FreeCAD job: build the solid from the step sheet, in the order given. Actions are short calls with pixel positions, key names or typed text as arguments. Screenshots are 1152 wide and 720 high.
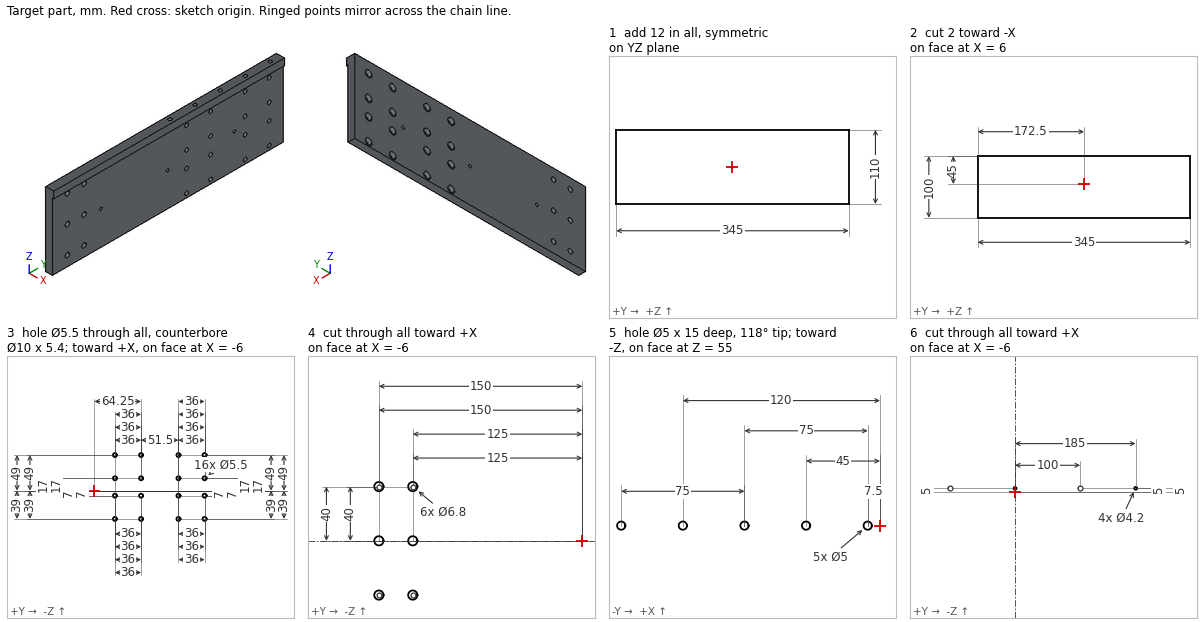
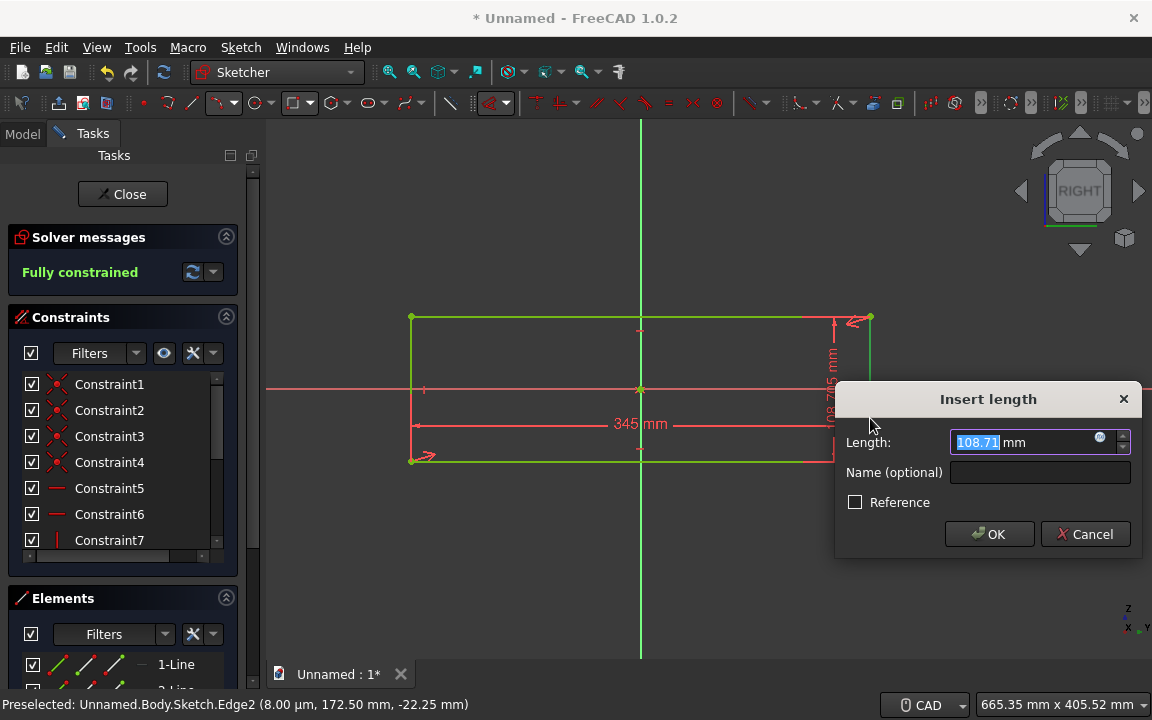
text(110)
key(Return)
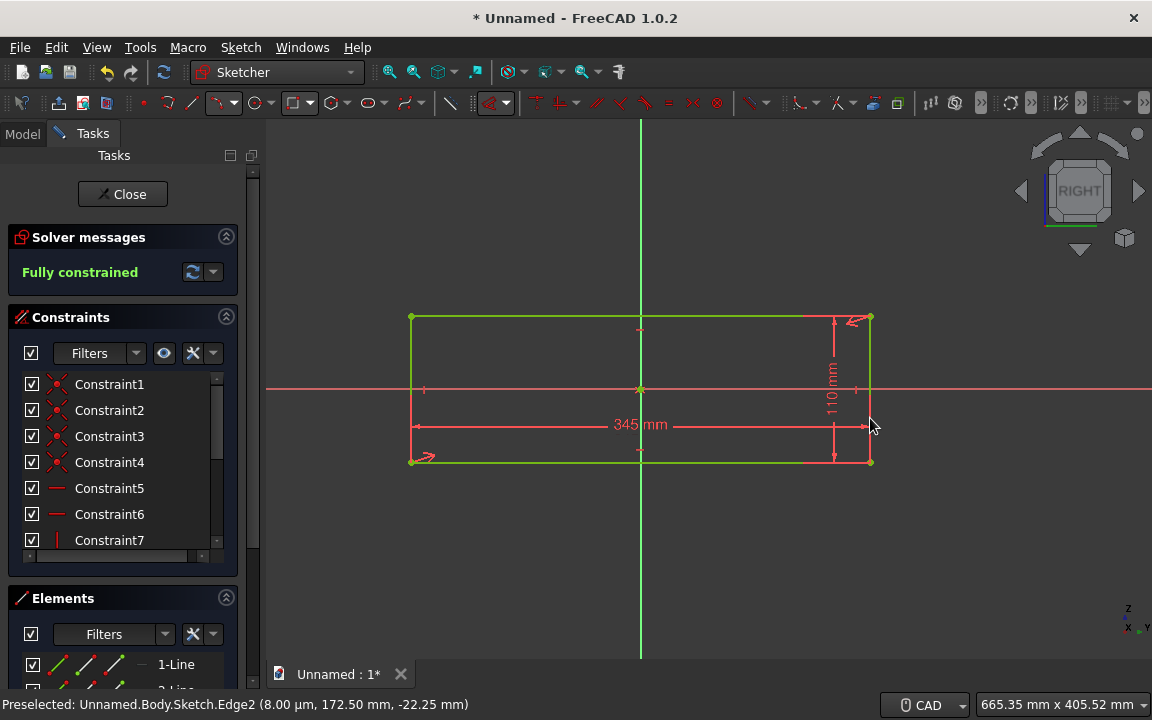
click(123, 194)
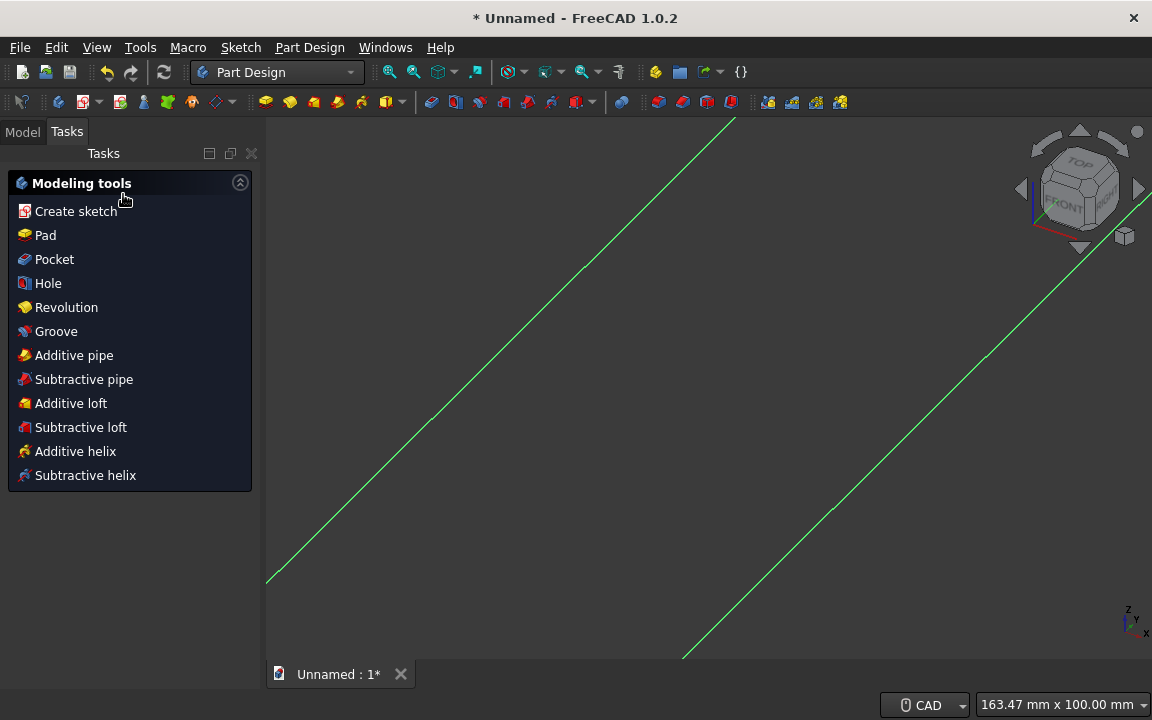
click(266, 102)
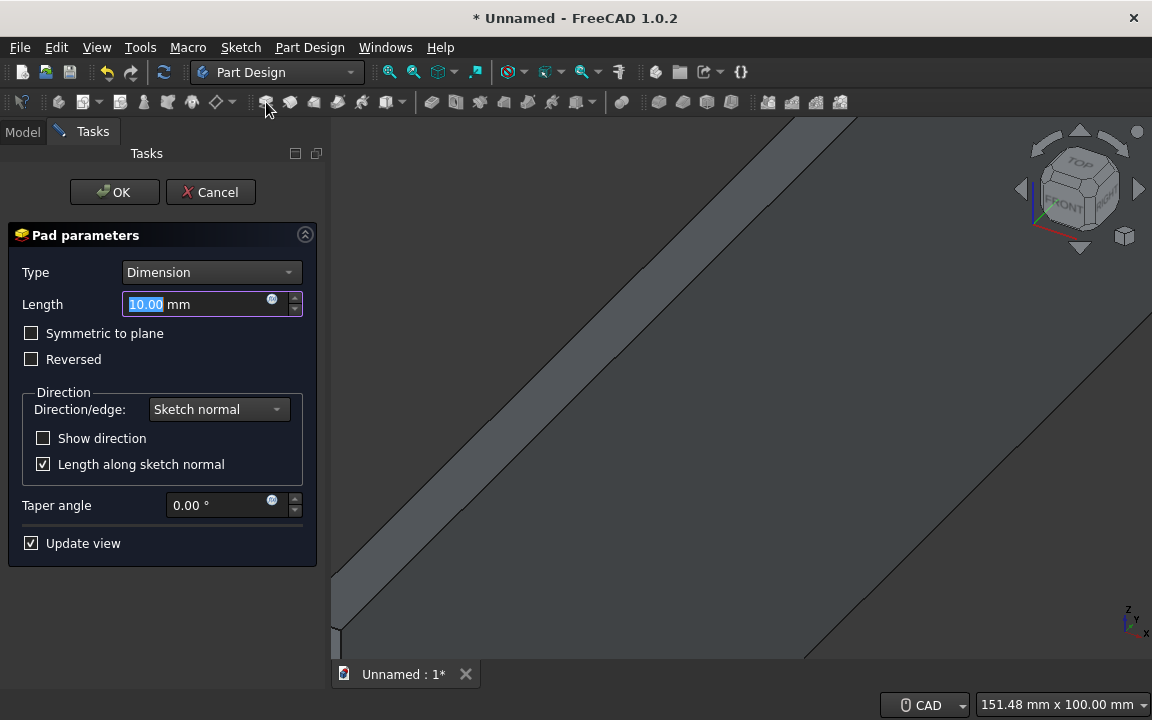
text(12)
key(Tab)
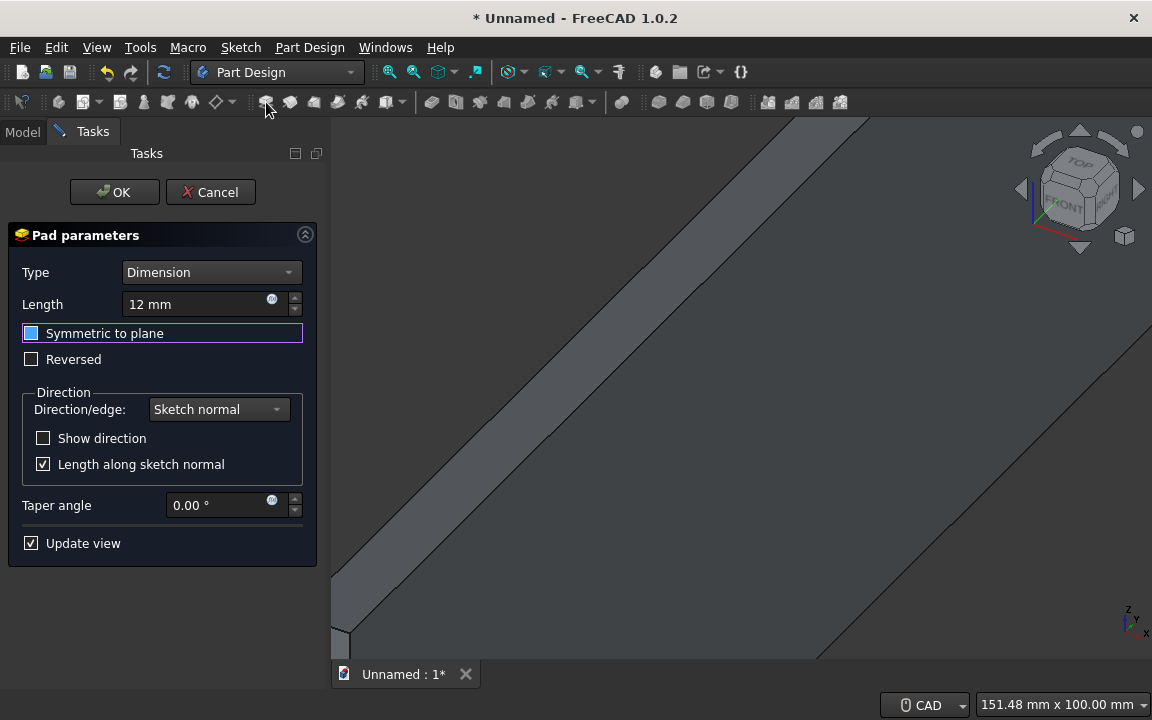
click(30, 333)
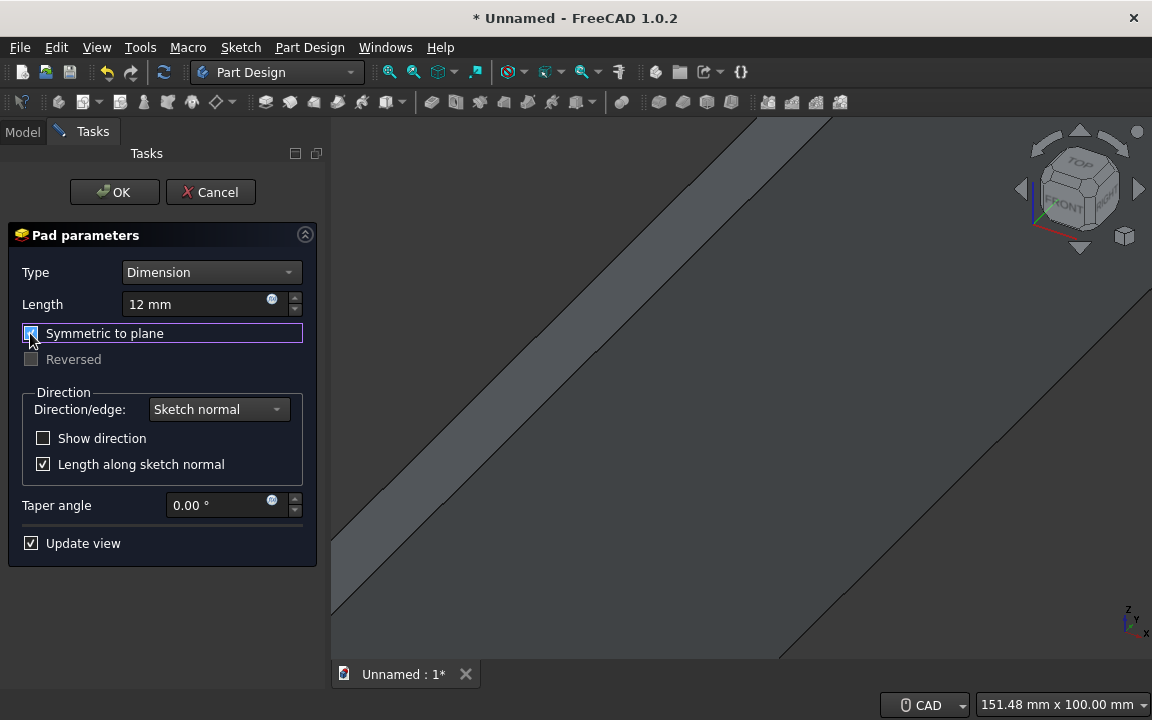
click(115, 192)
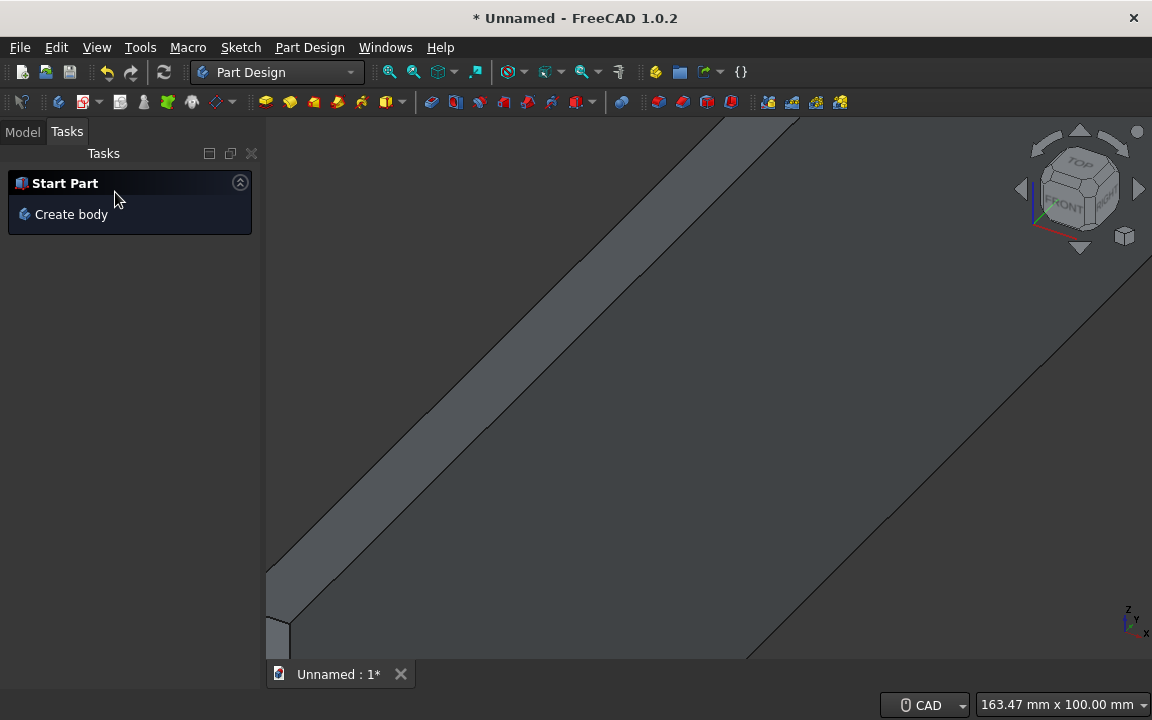
click(390, 72)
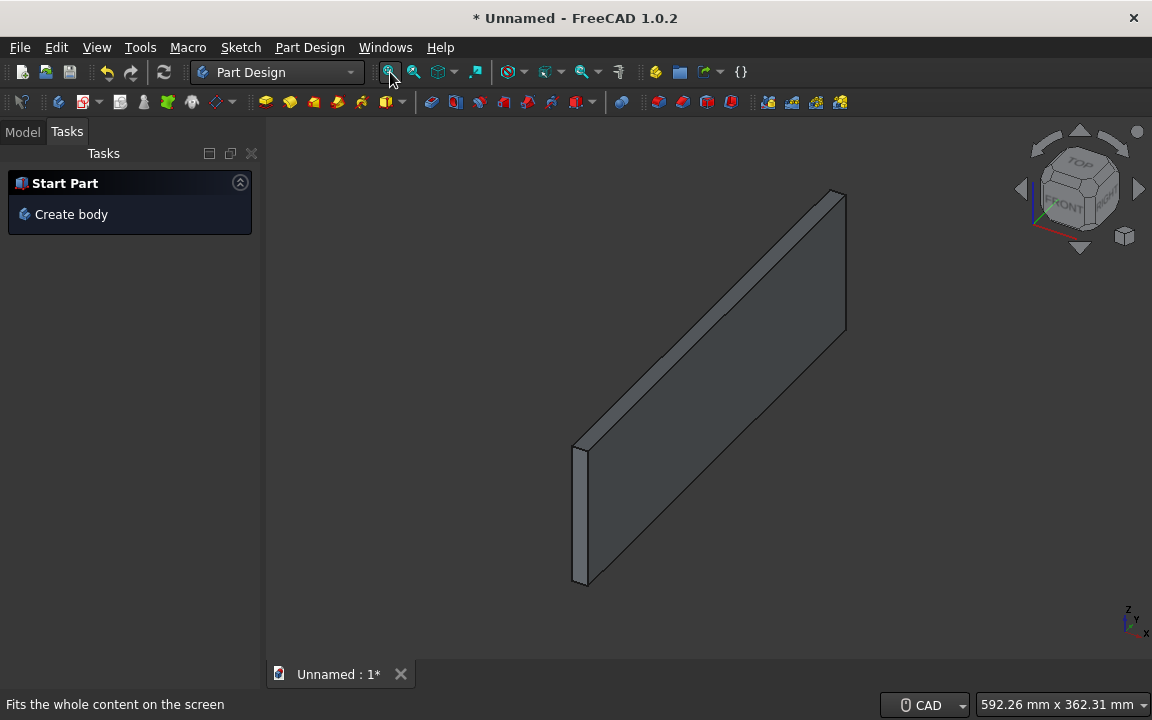
click(791, 316)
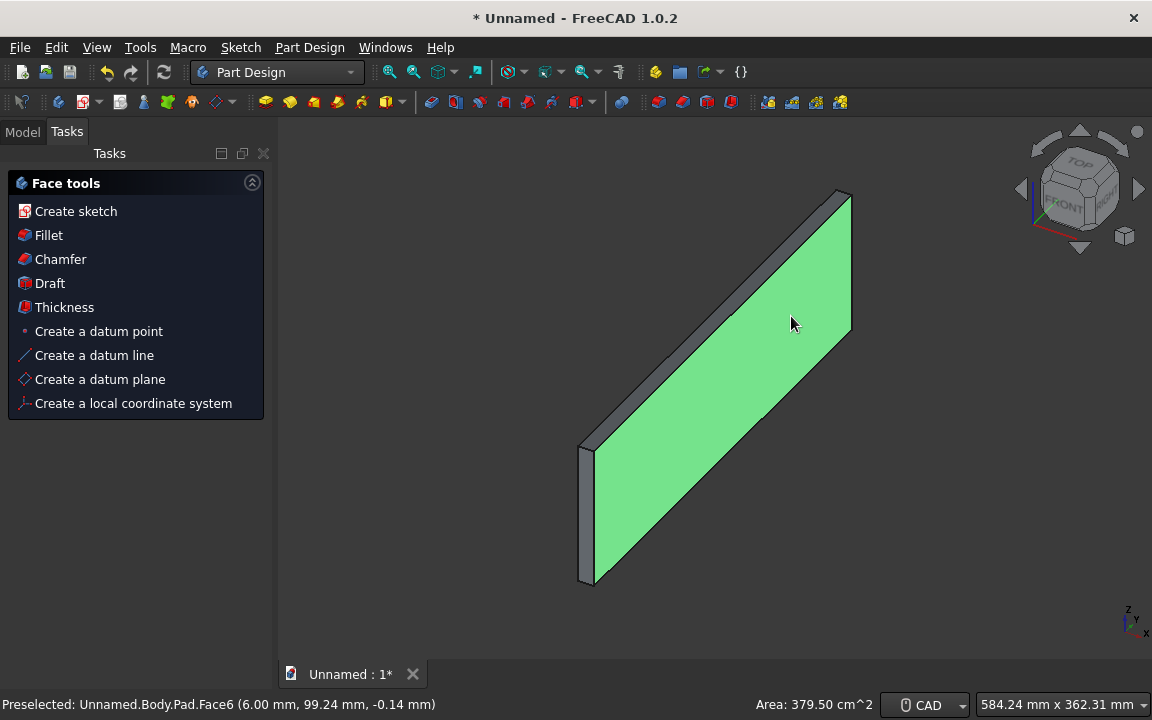
click(84, 102)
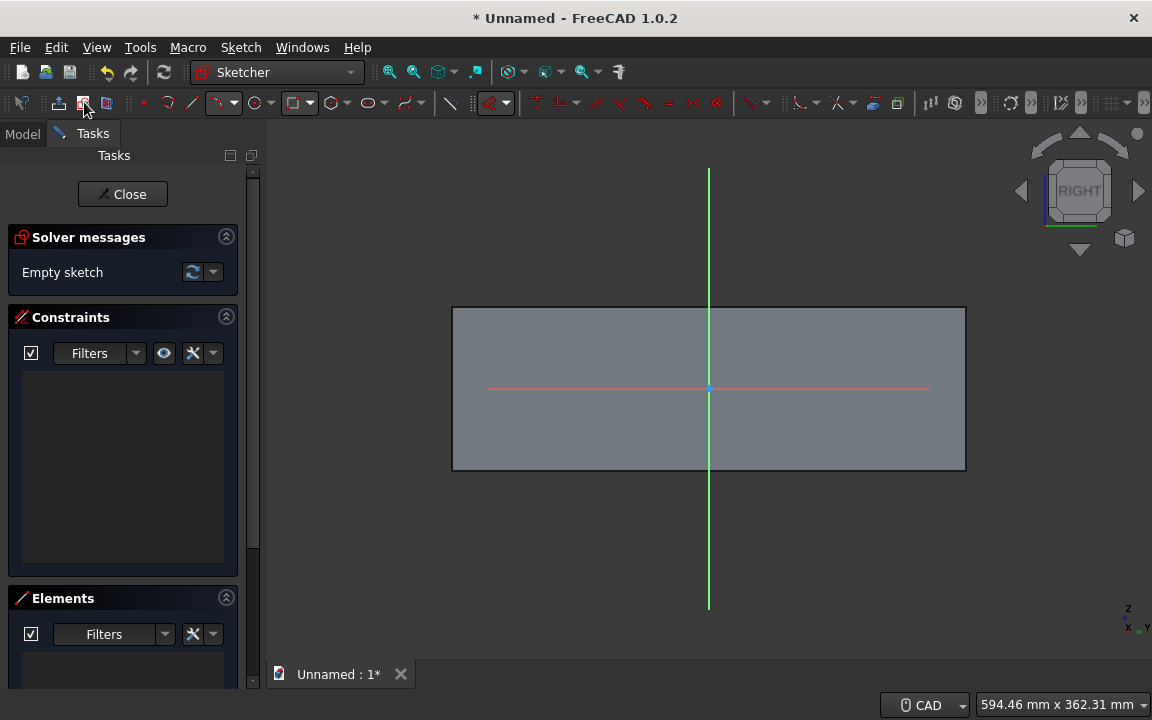
scroll(331, 355, down, 1)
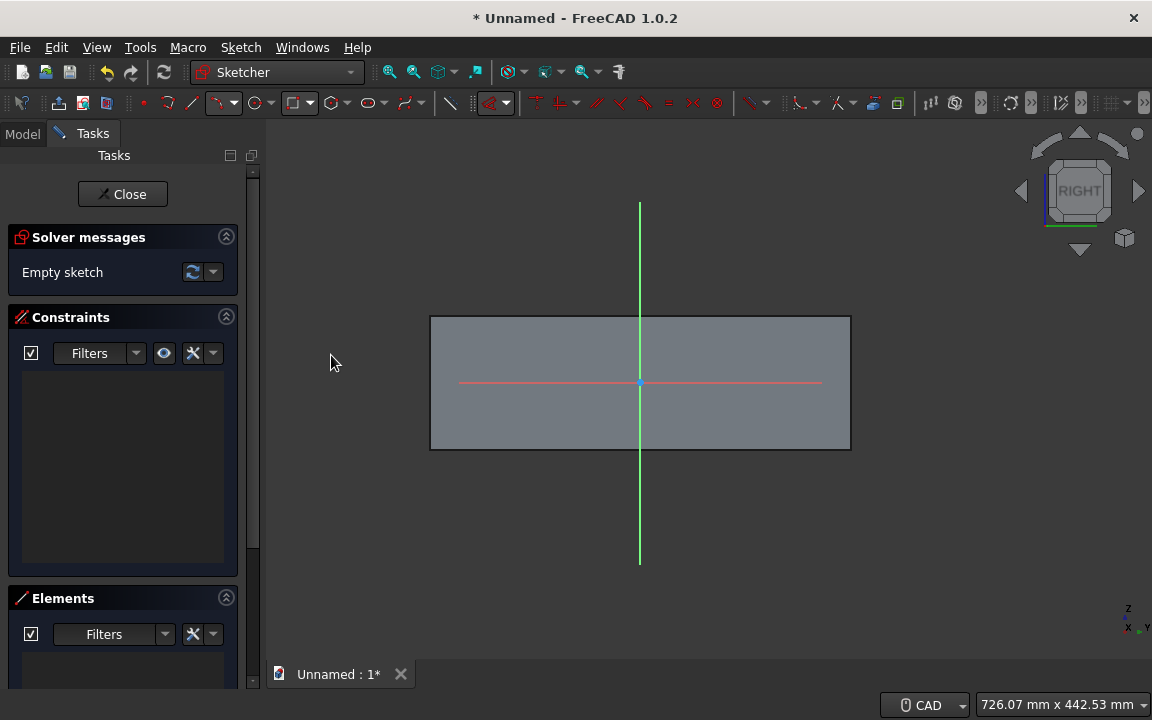
click(294, 104)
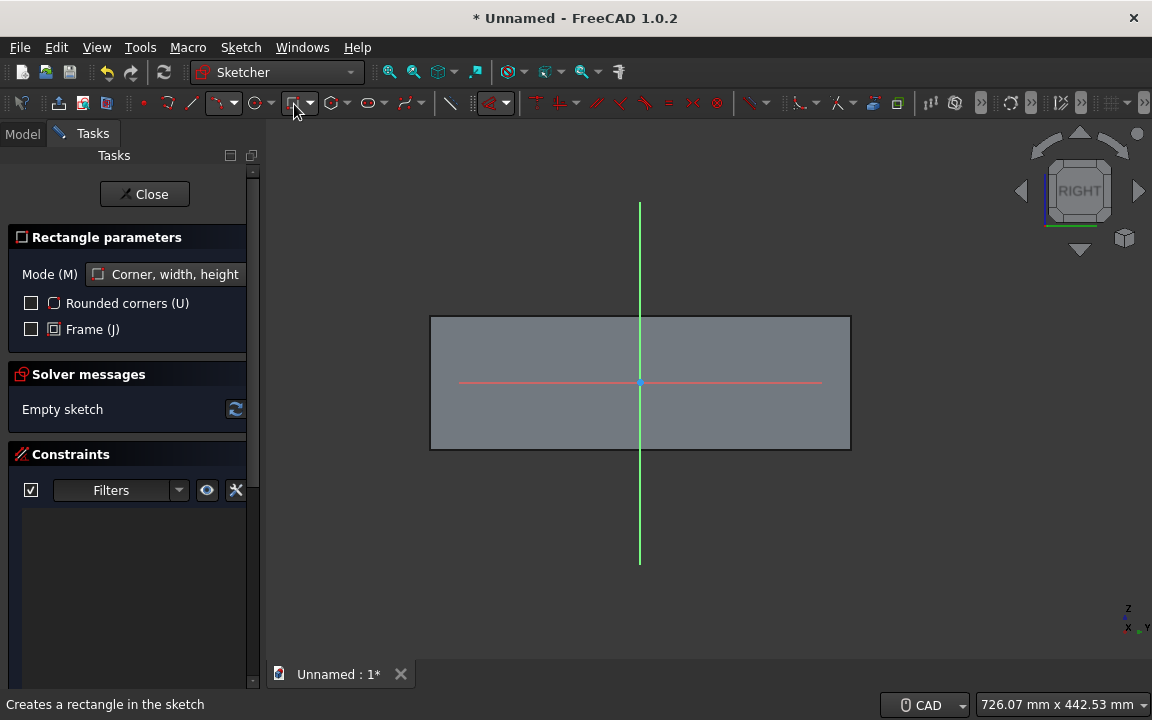
click(430, 328)
click(851, 450)
key(Escape)